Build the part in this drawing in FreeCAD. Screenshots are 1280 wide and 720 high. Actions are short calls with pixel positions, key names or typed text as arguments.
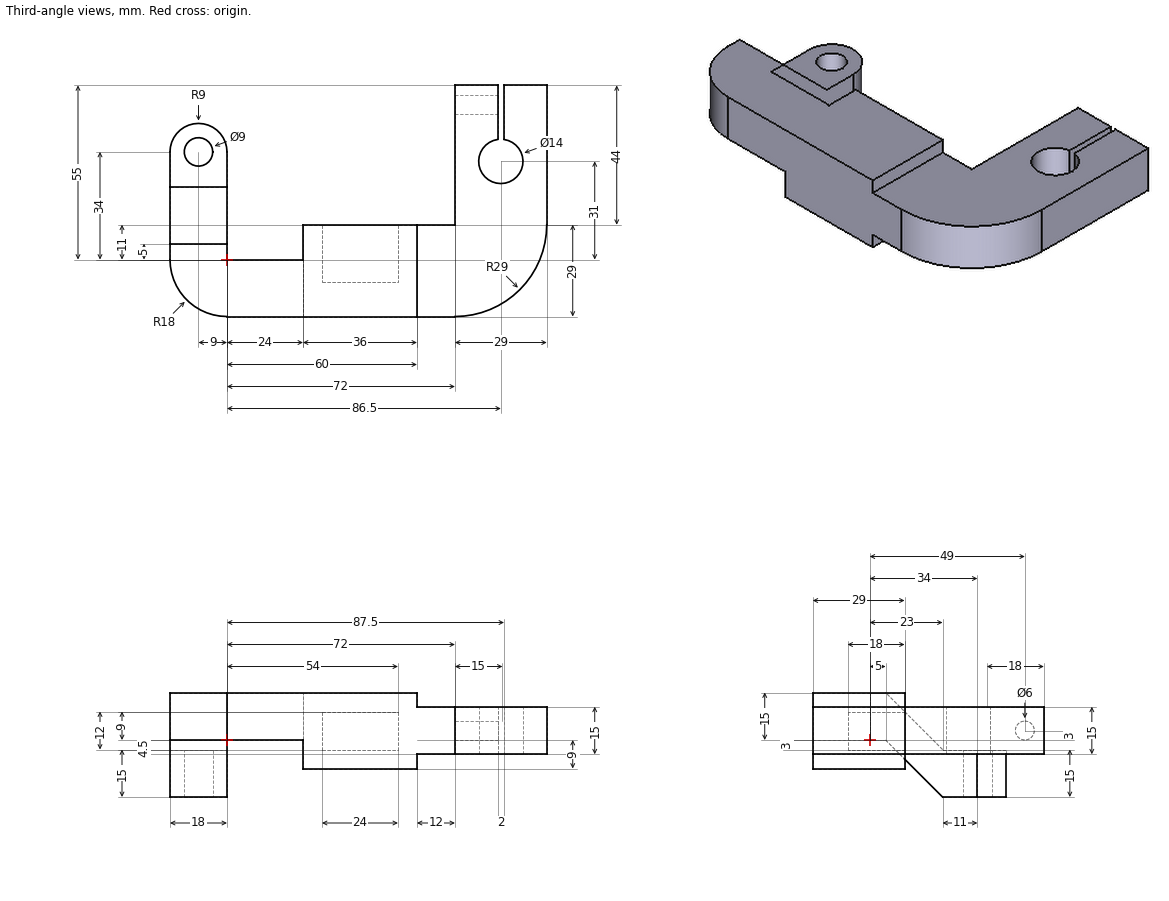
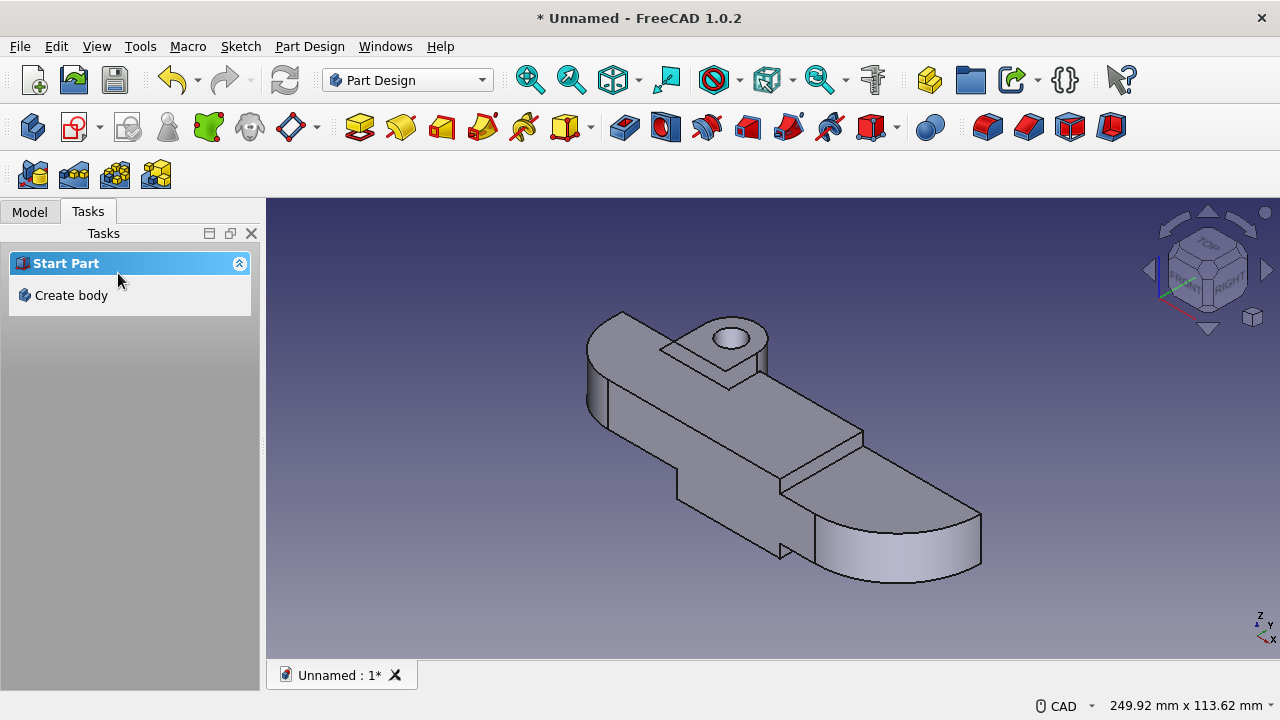
click(864, 493)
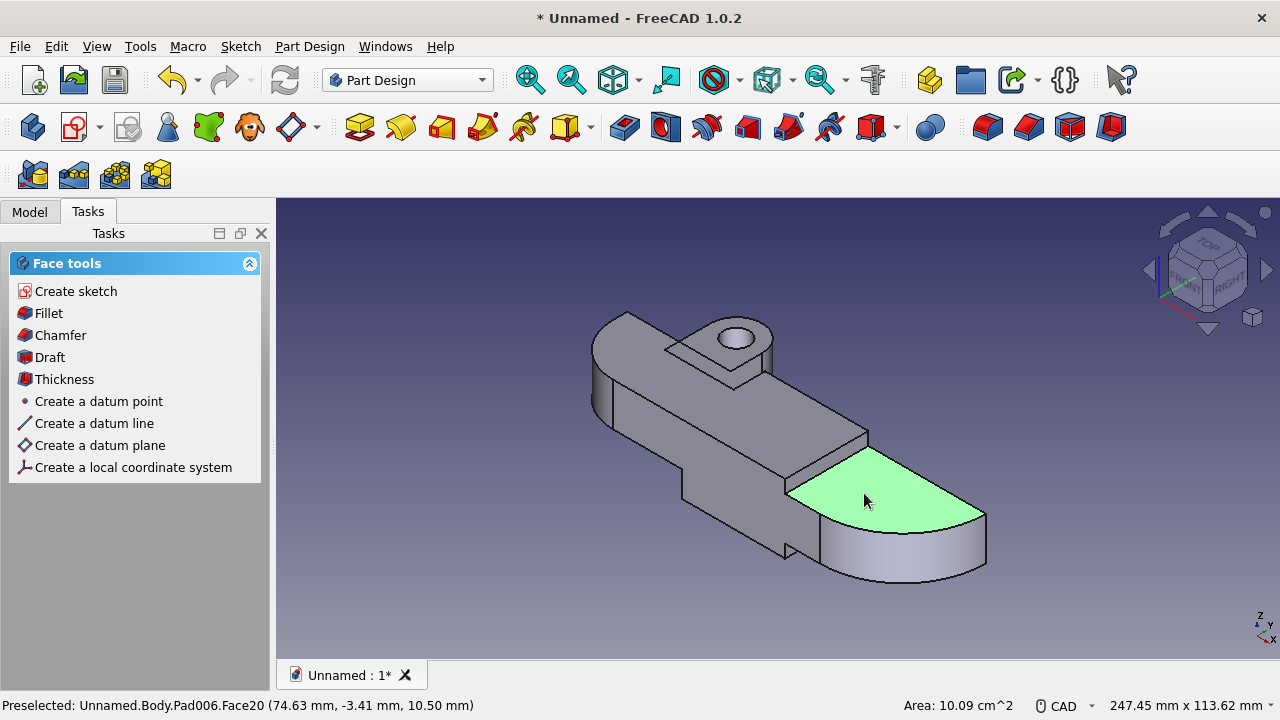
click(74, 128)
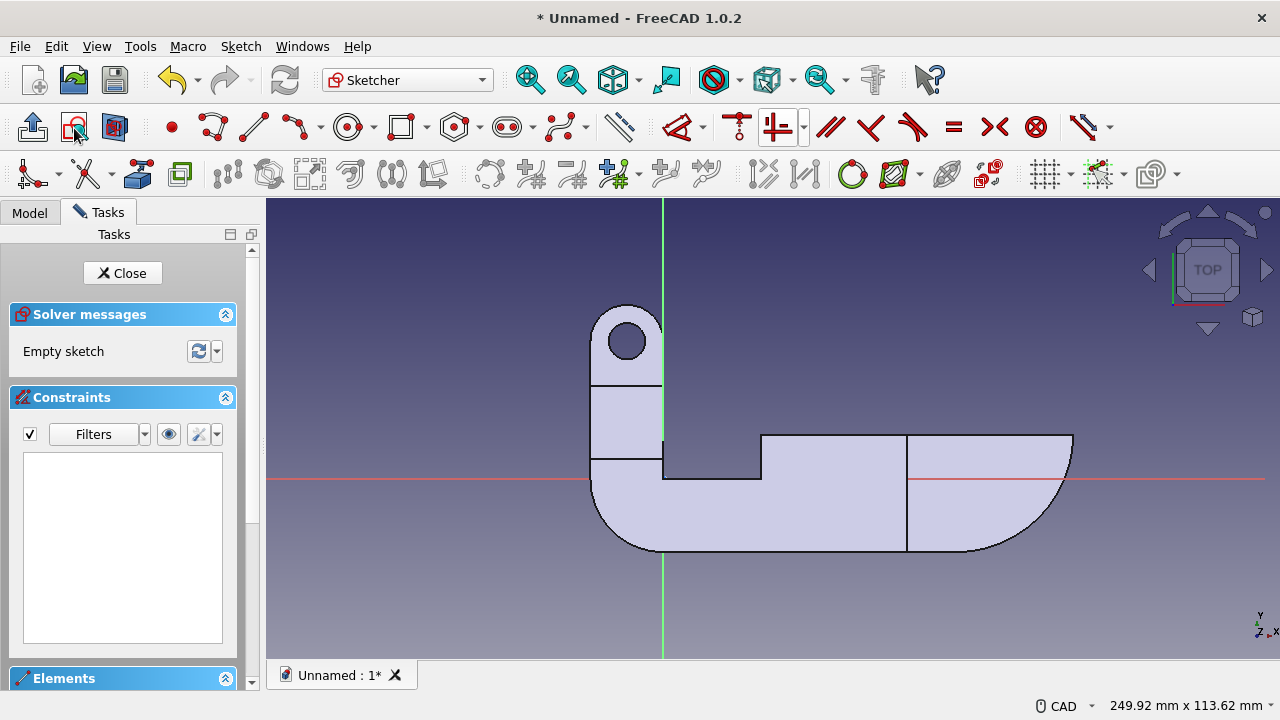
click(400, 128)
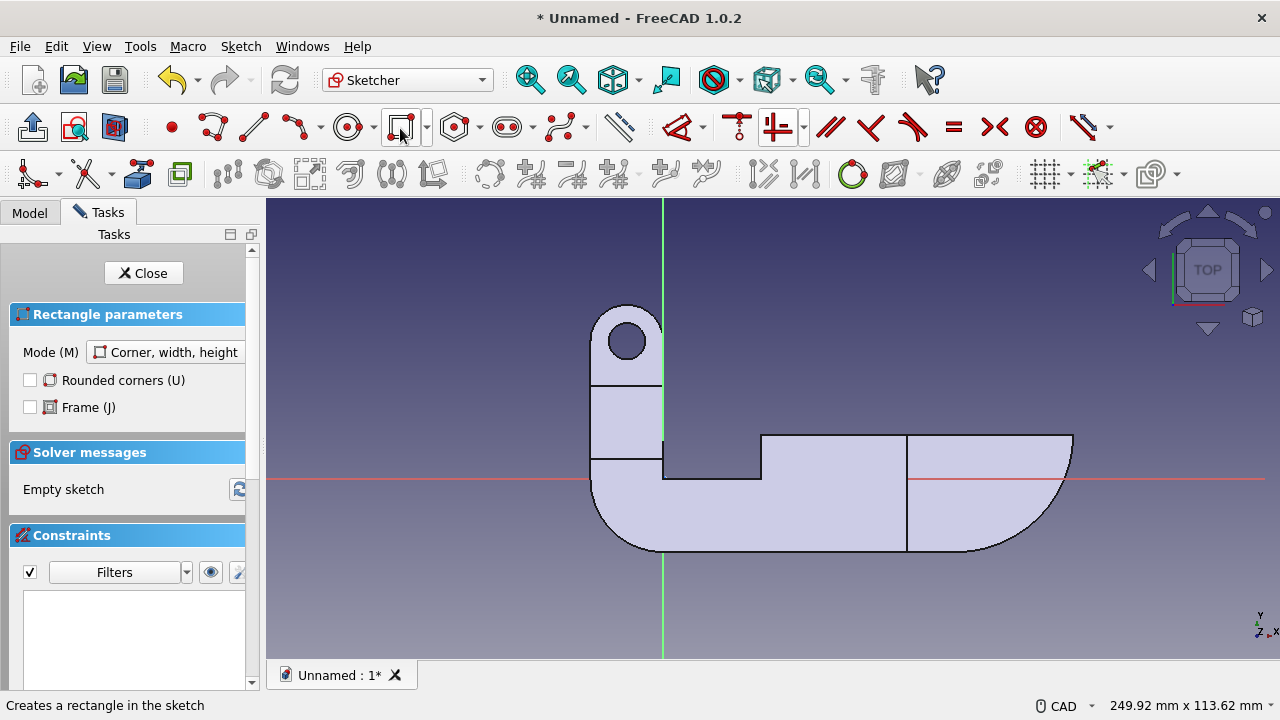
click(956, 256)
move(1073, 435)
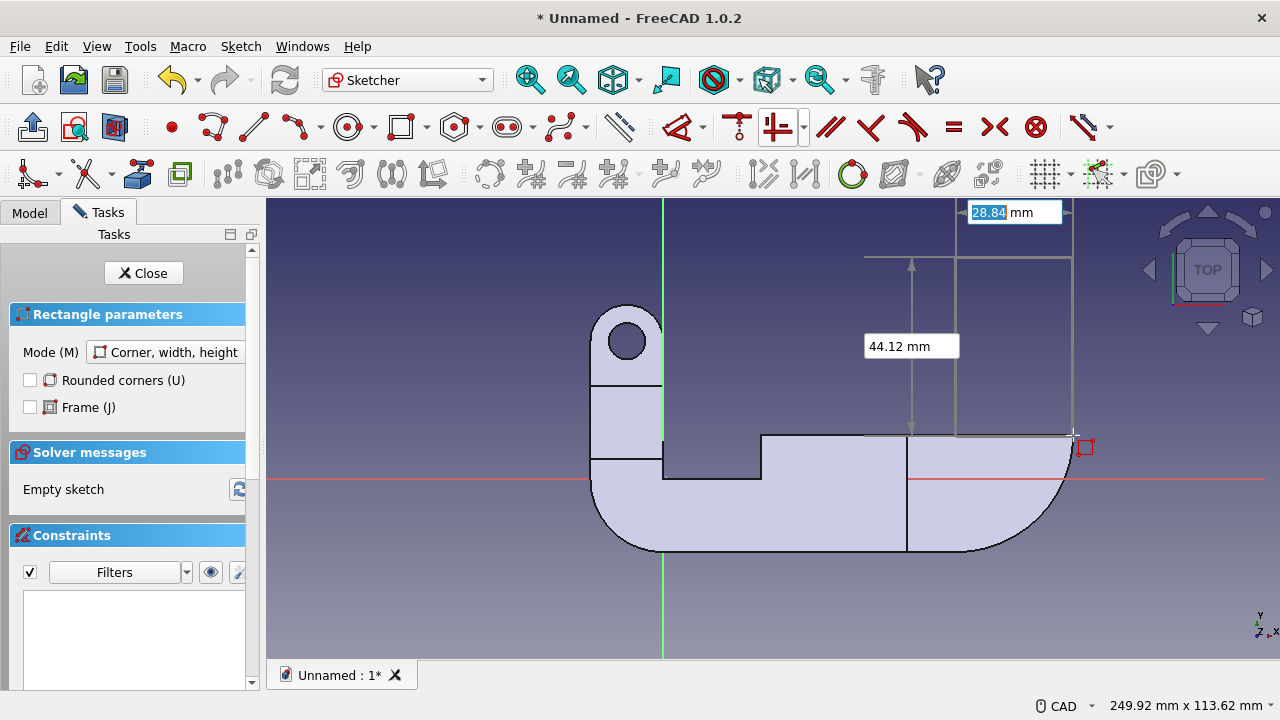
text(29)
key(Tab)
text(44)
key(Return)
key(Escape)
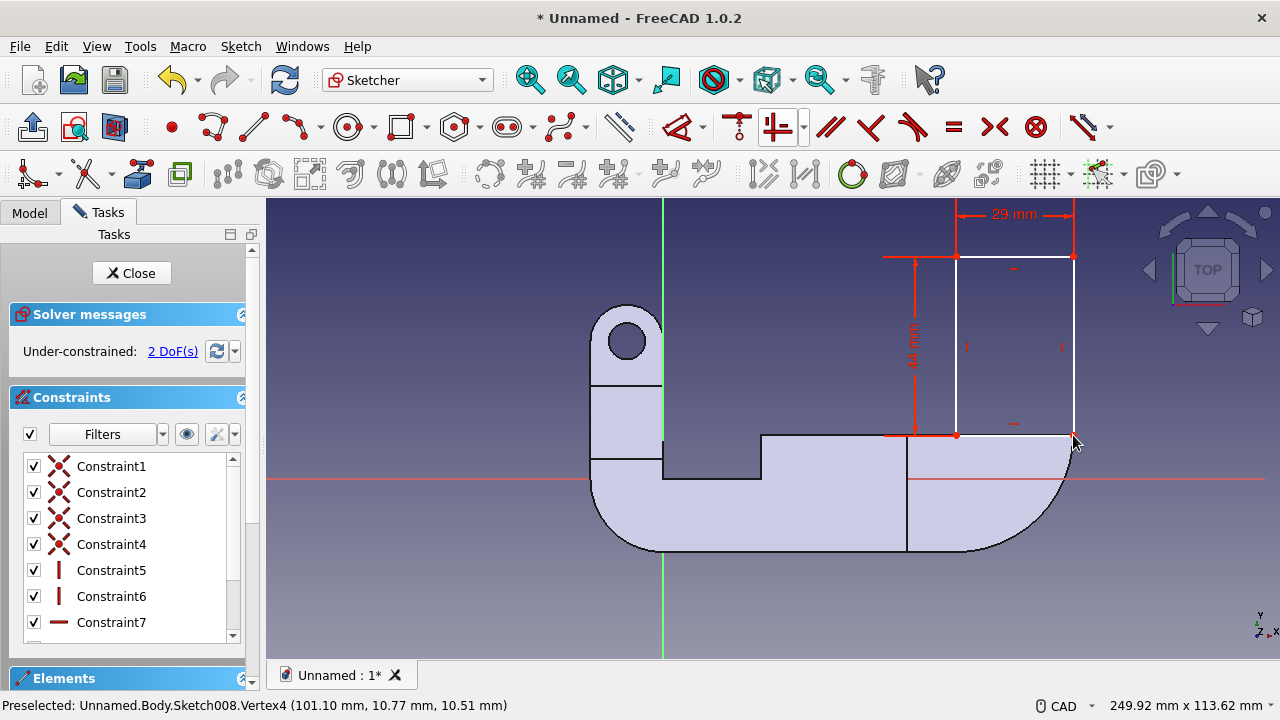
click(676, 128)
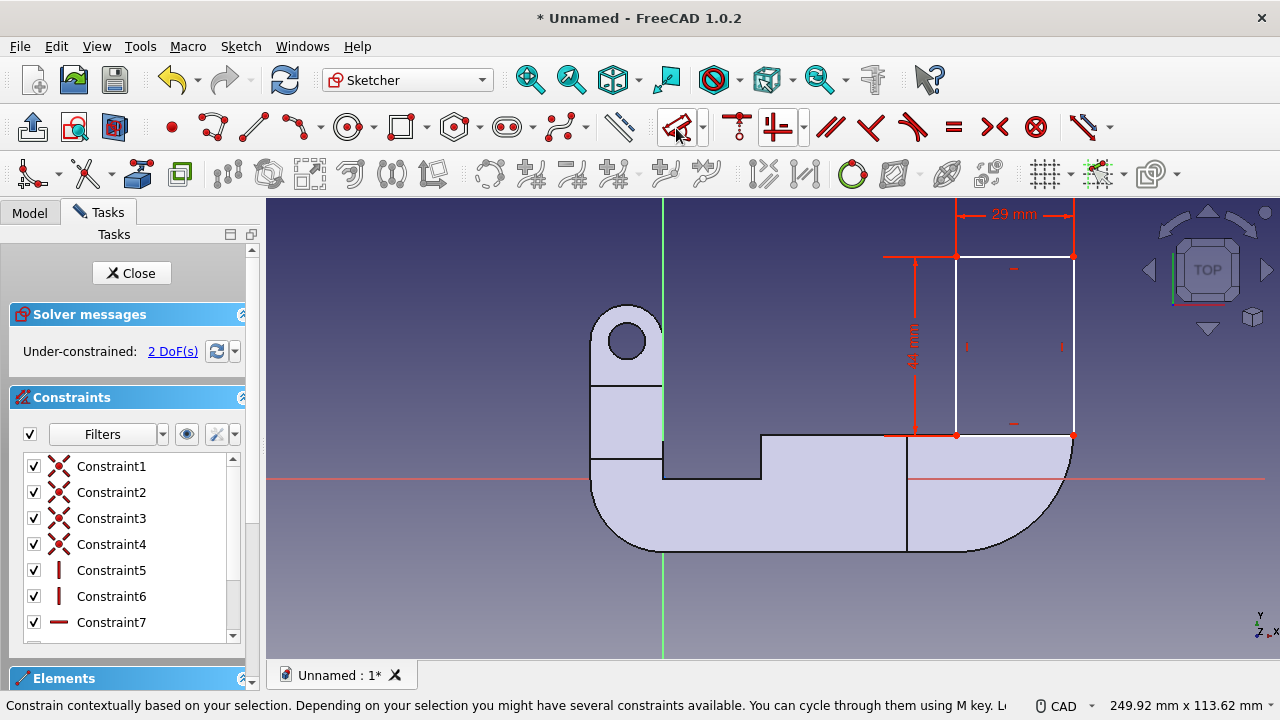
click(956, 257)
click(810, 513)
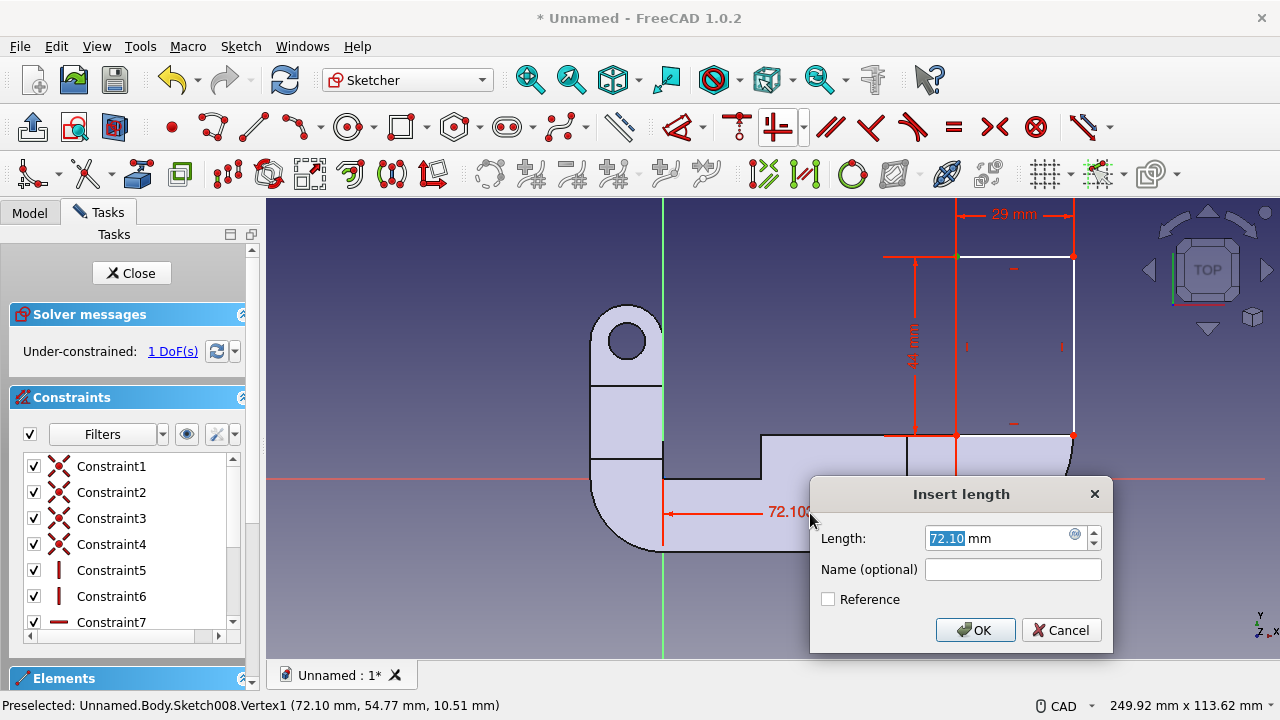
text(72)
key(Return)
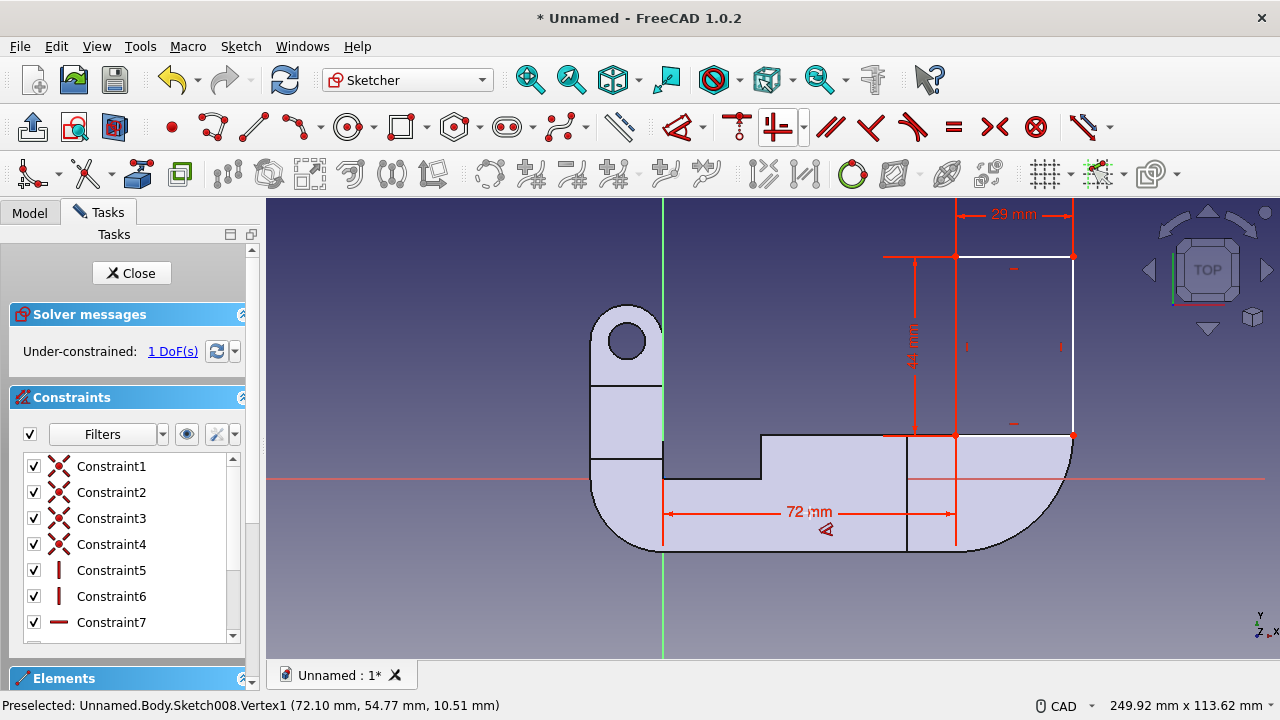
click(956, 257)
click(629, 368)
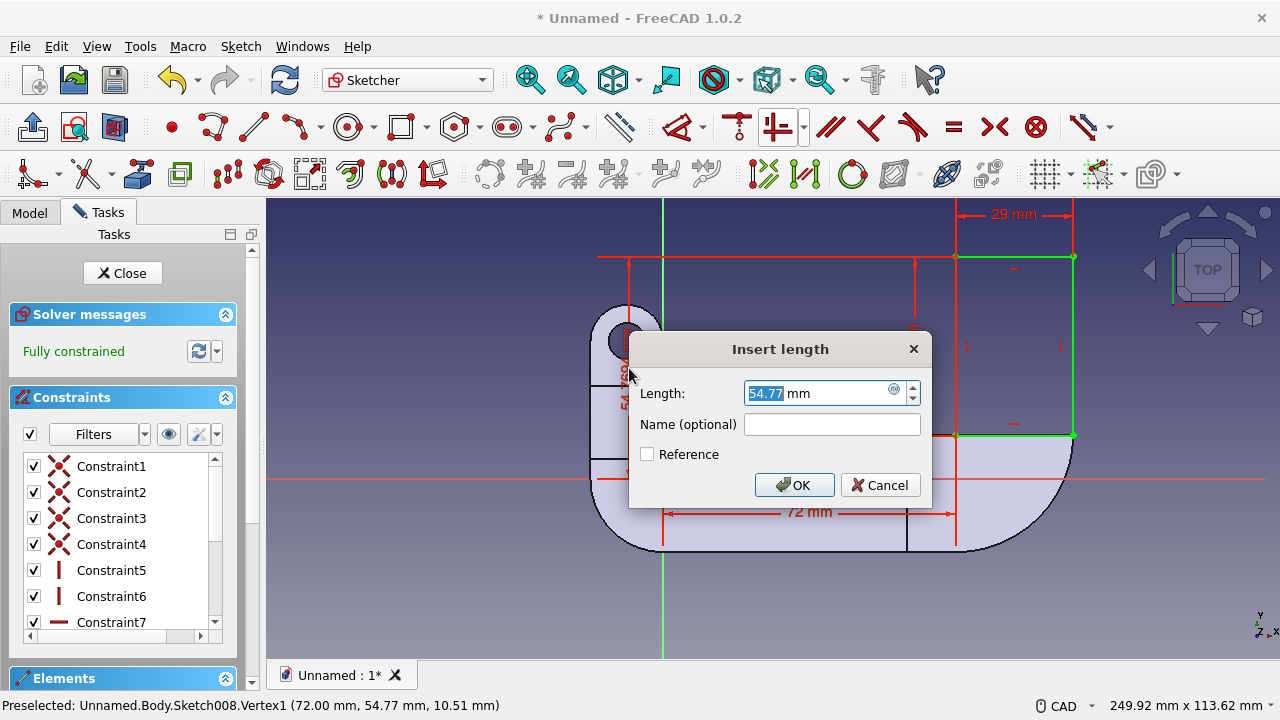
text(55)
key(Return)
key(Escape)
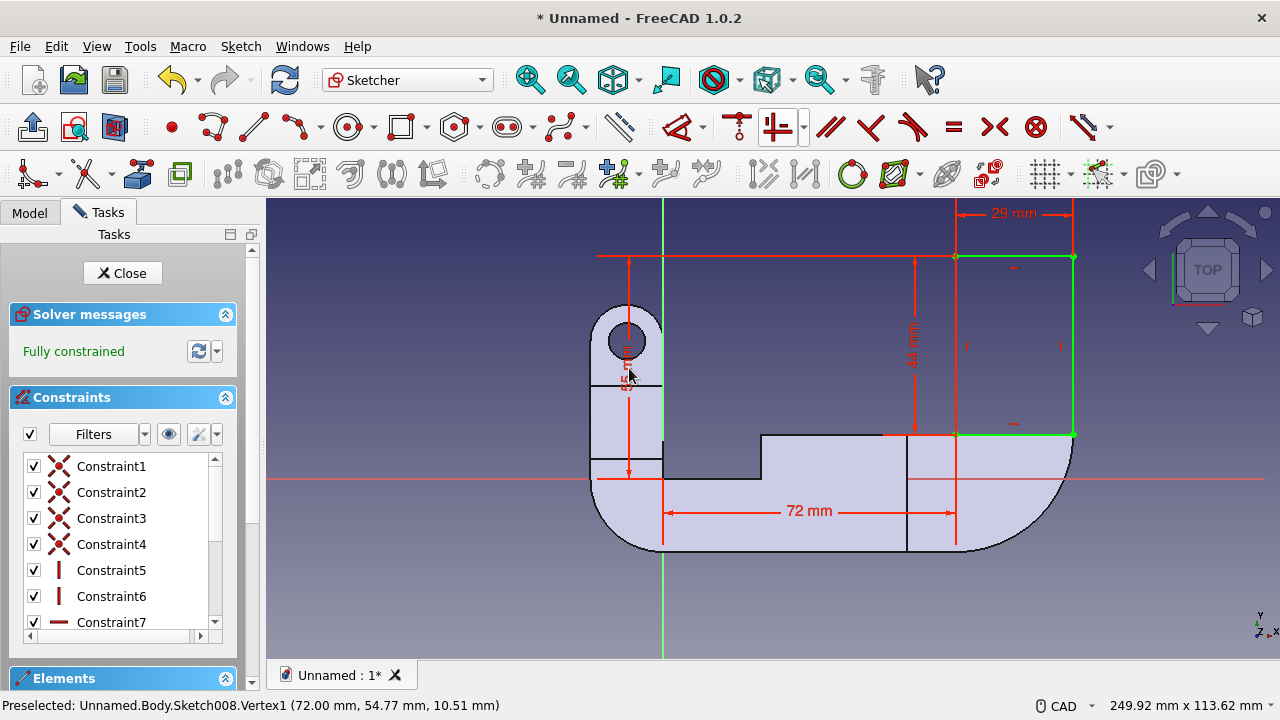
click(123, 273)